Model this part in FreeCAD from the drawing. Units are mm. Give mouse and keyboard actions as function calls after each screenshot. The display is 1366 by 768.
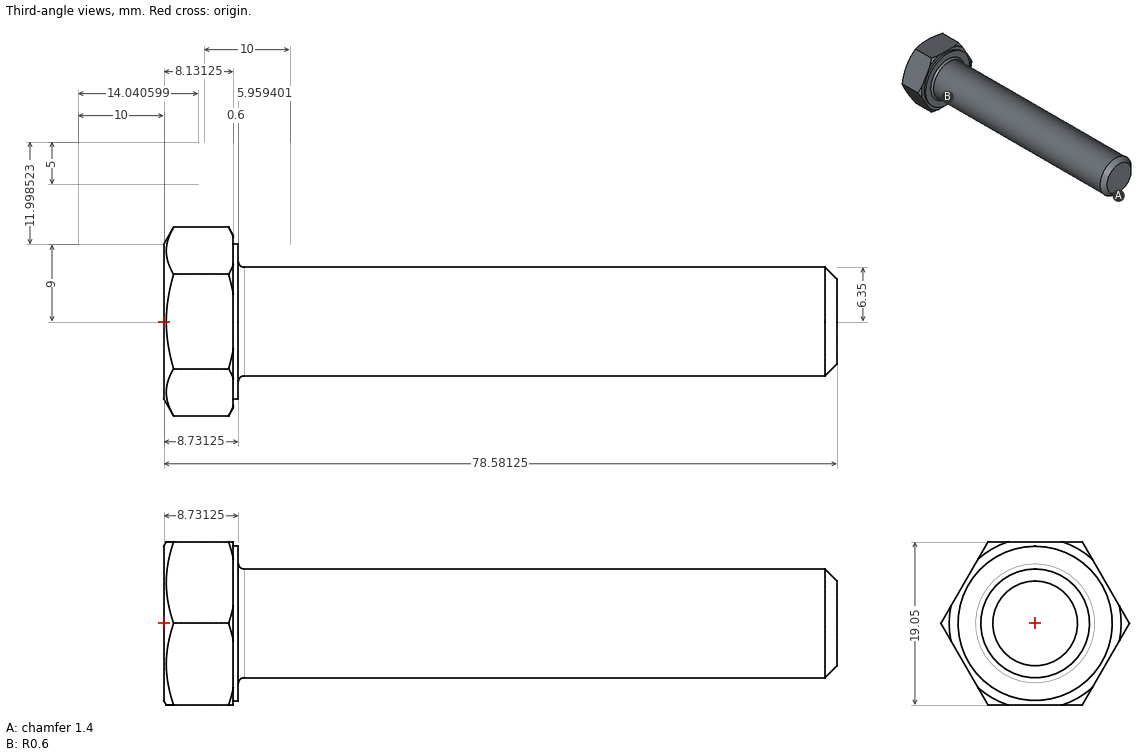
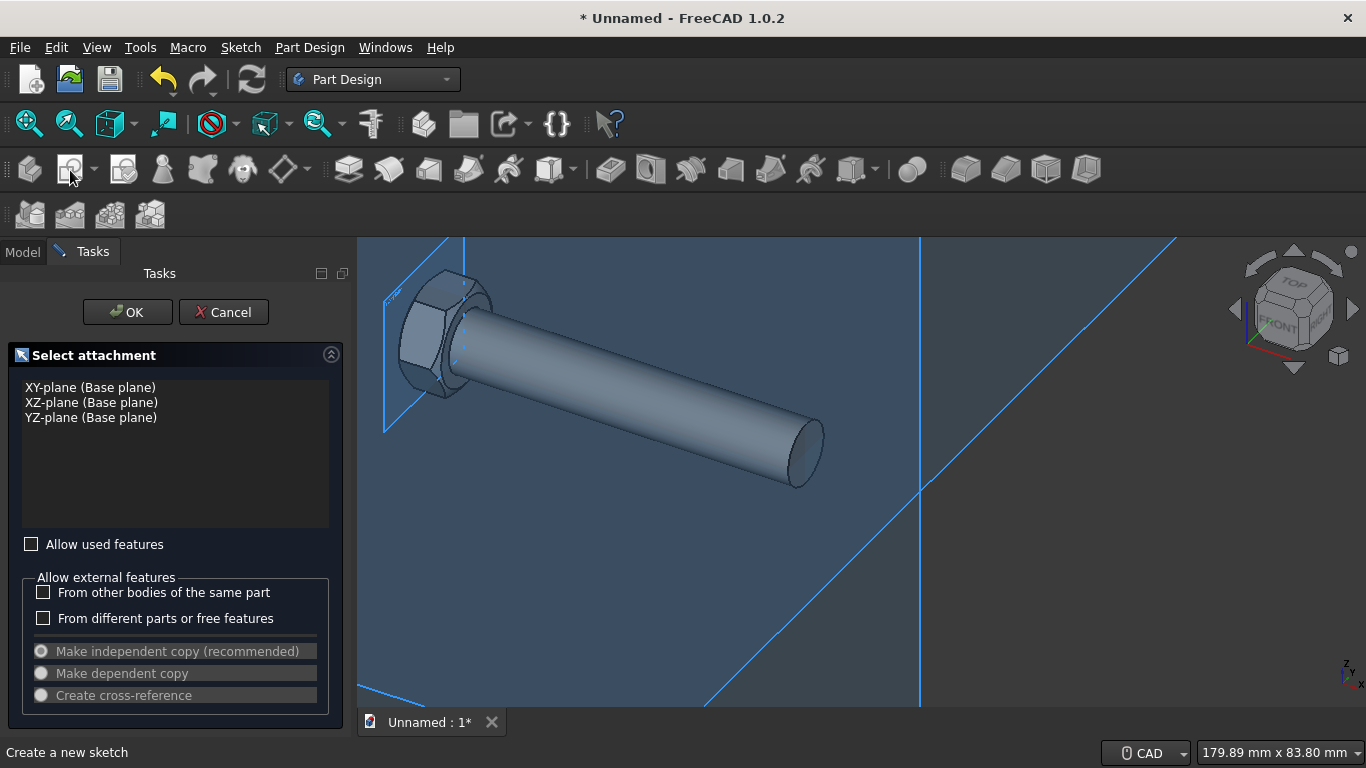
click(82, 388)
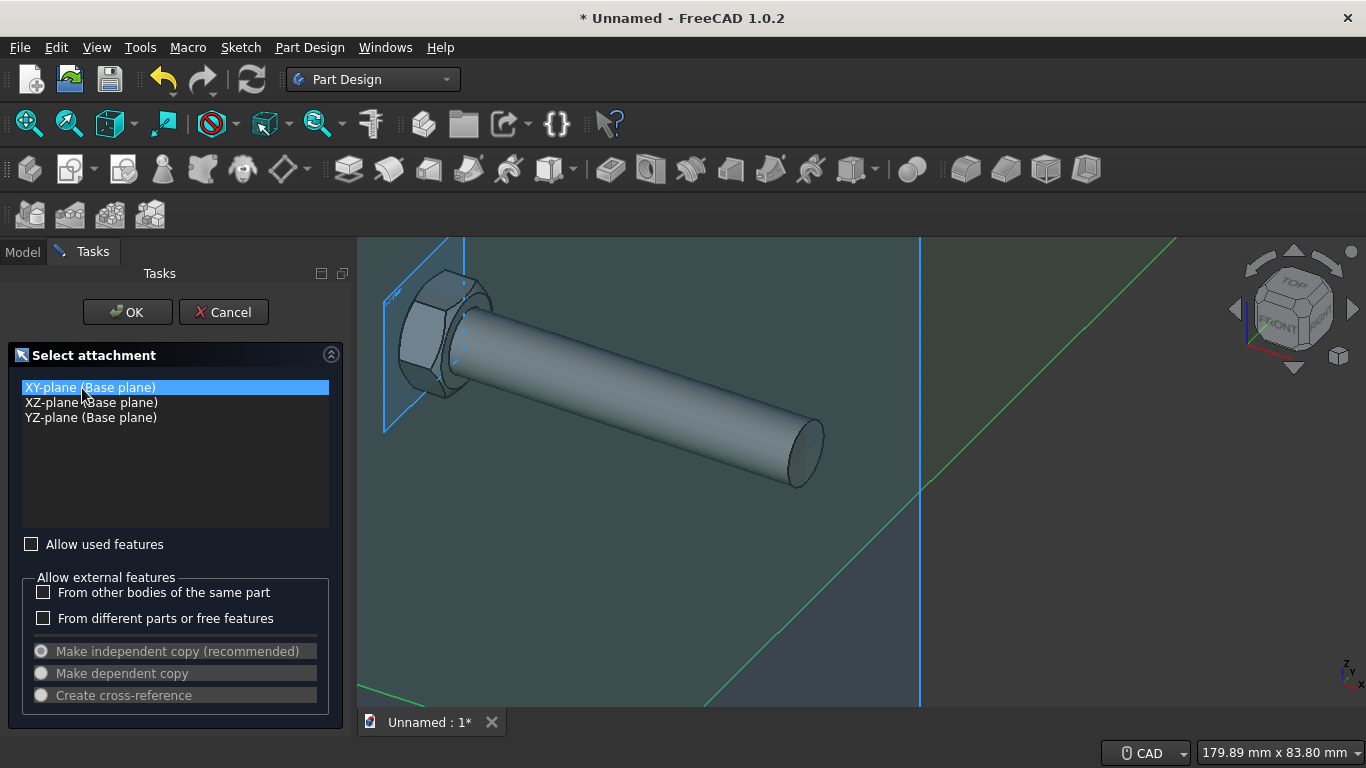
click(128, 312)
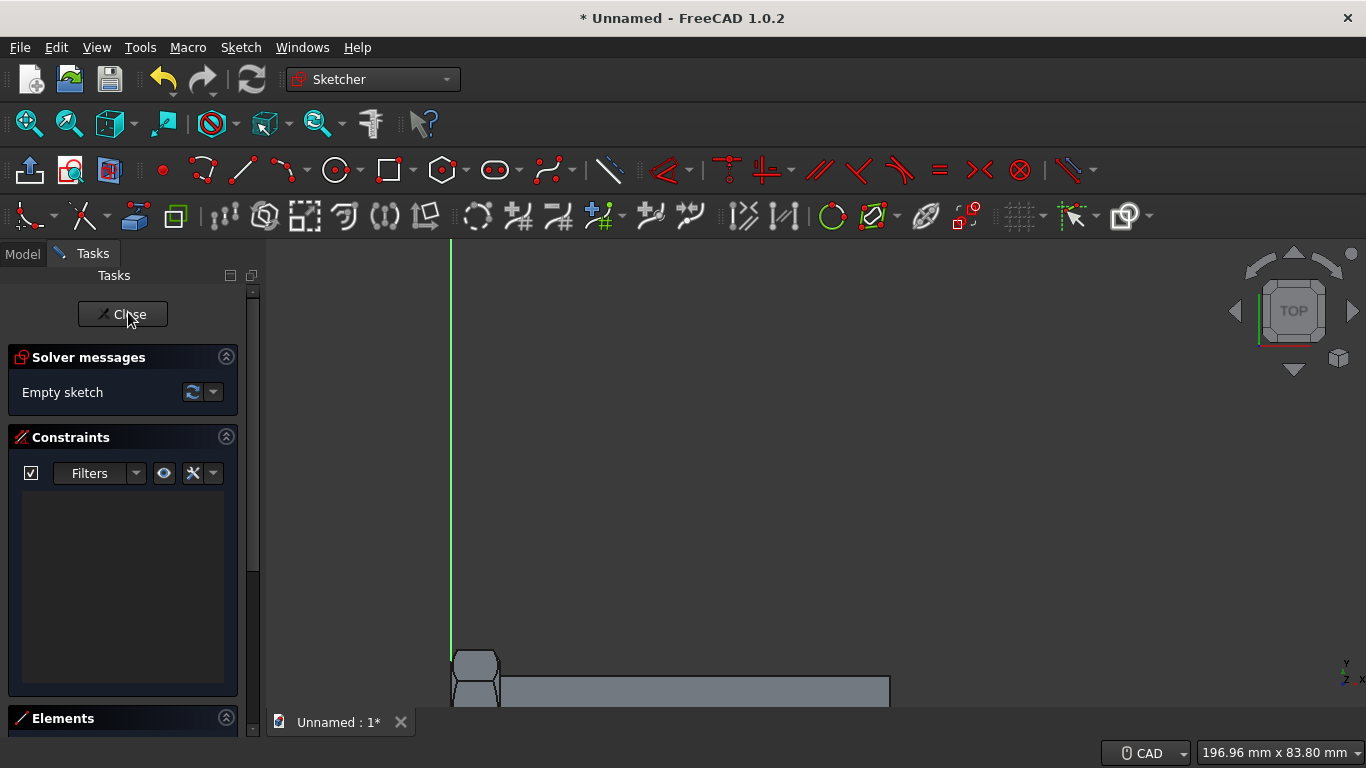
click(110, 170)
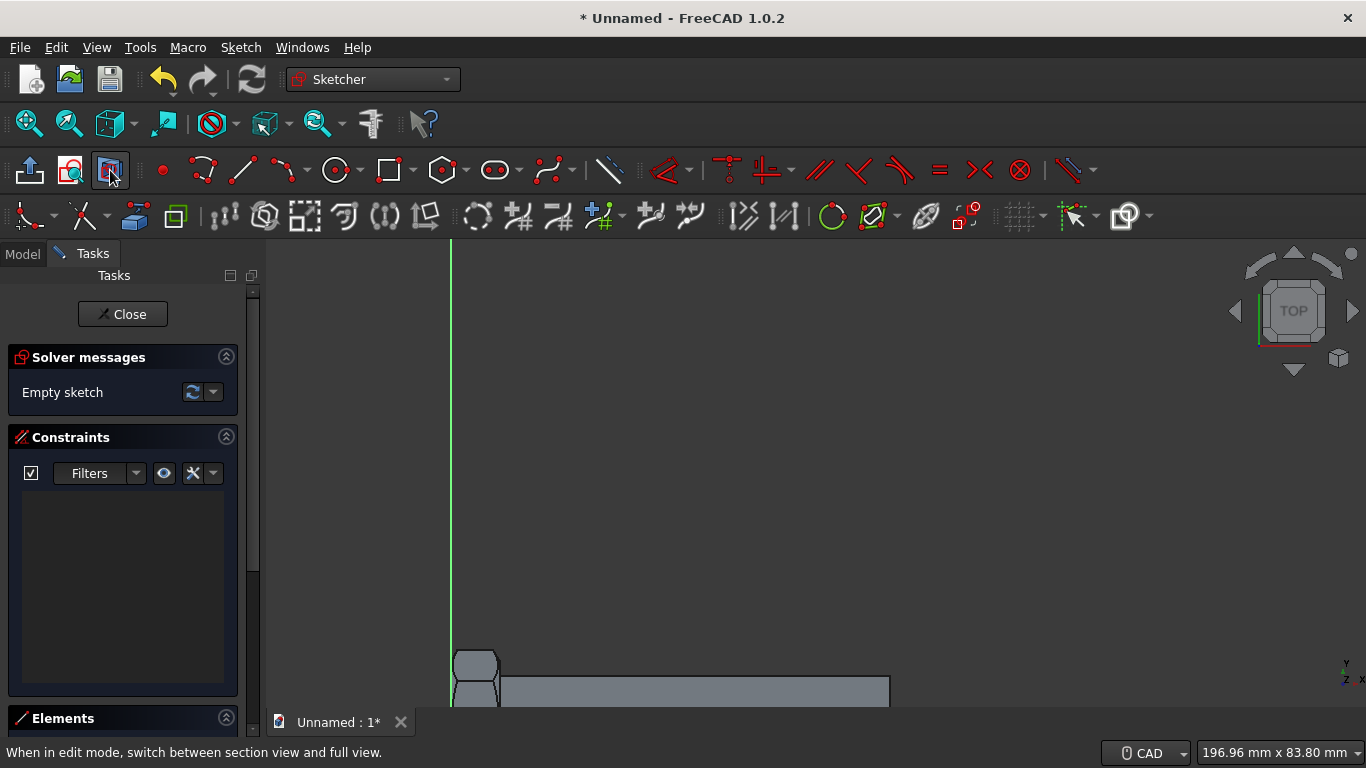
scroll(748, 473, down, 5)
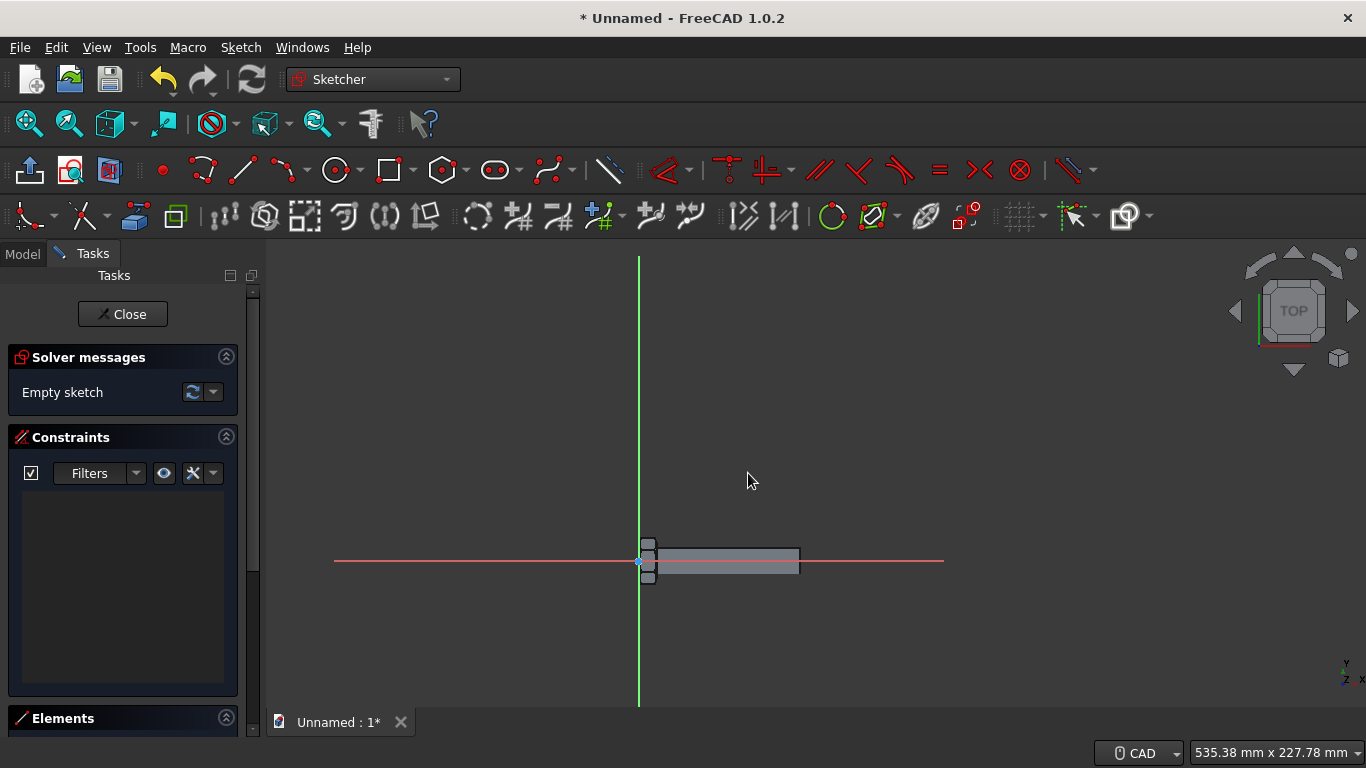
scroll(632, 550, up, 10)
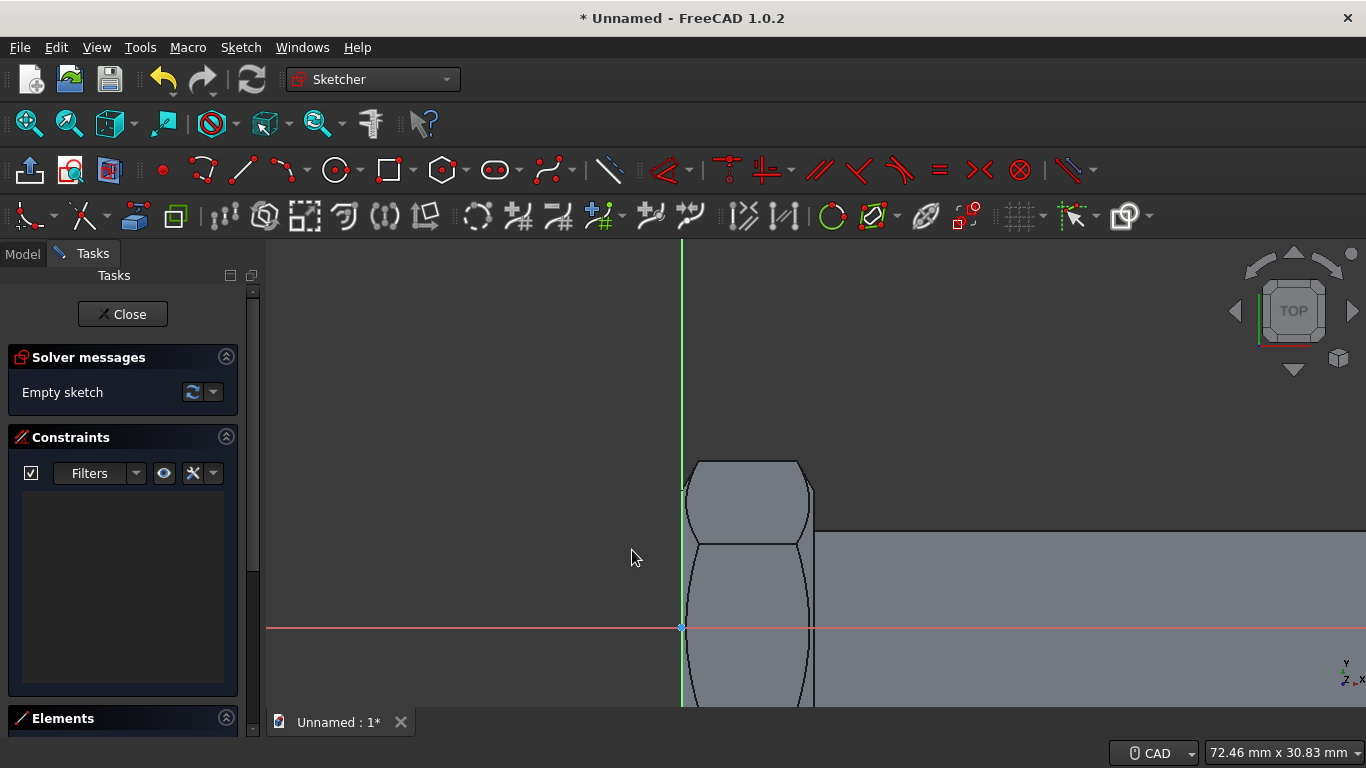
click(390, 170)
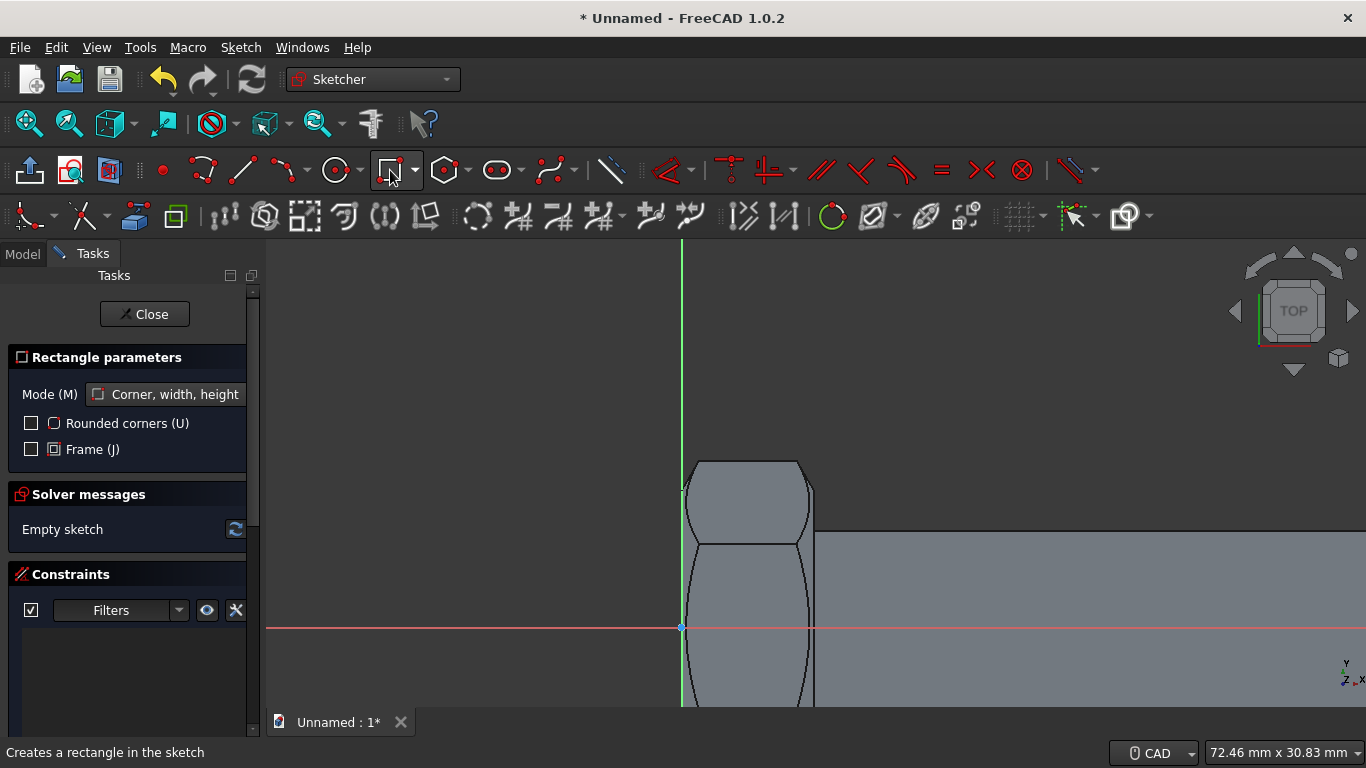
scroll(805, 309, up, 3)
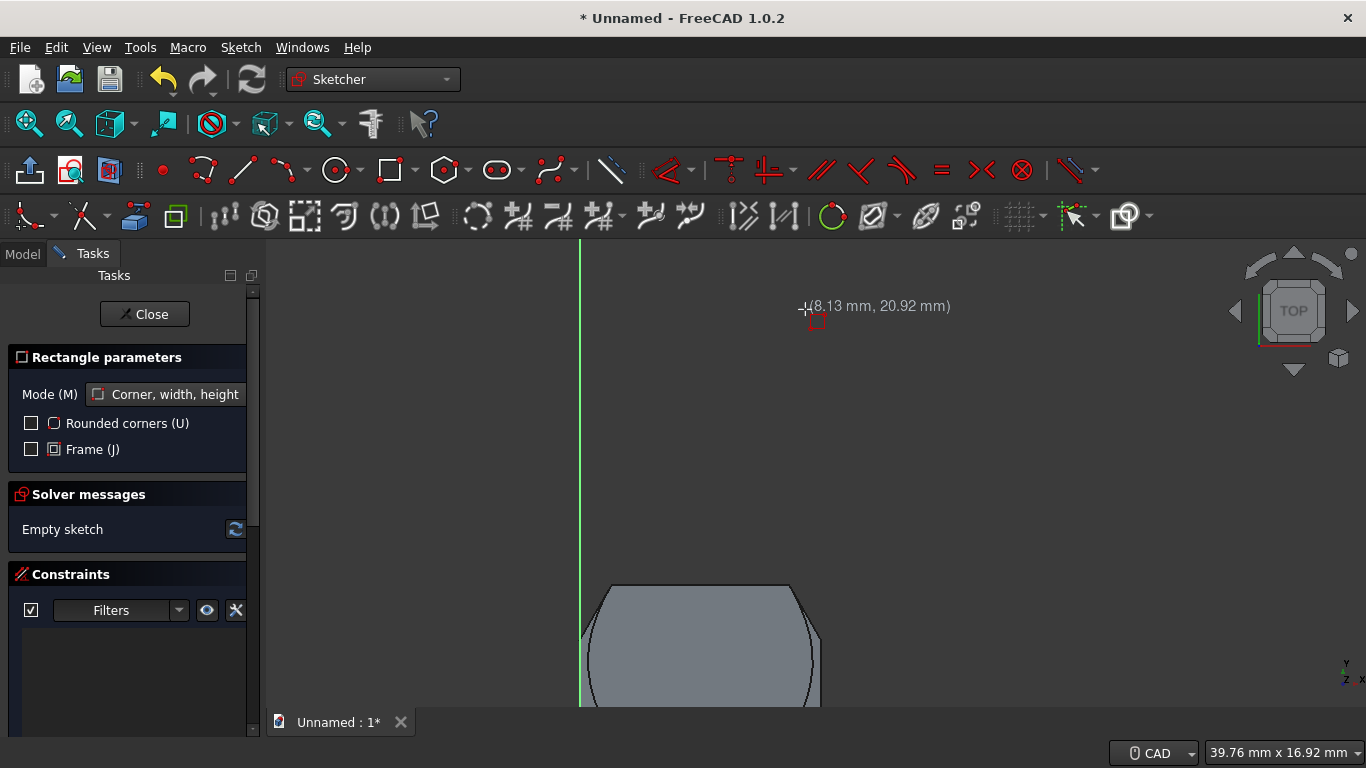
click(805, 308)
move(821, 640)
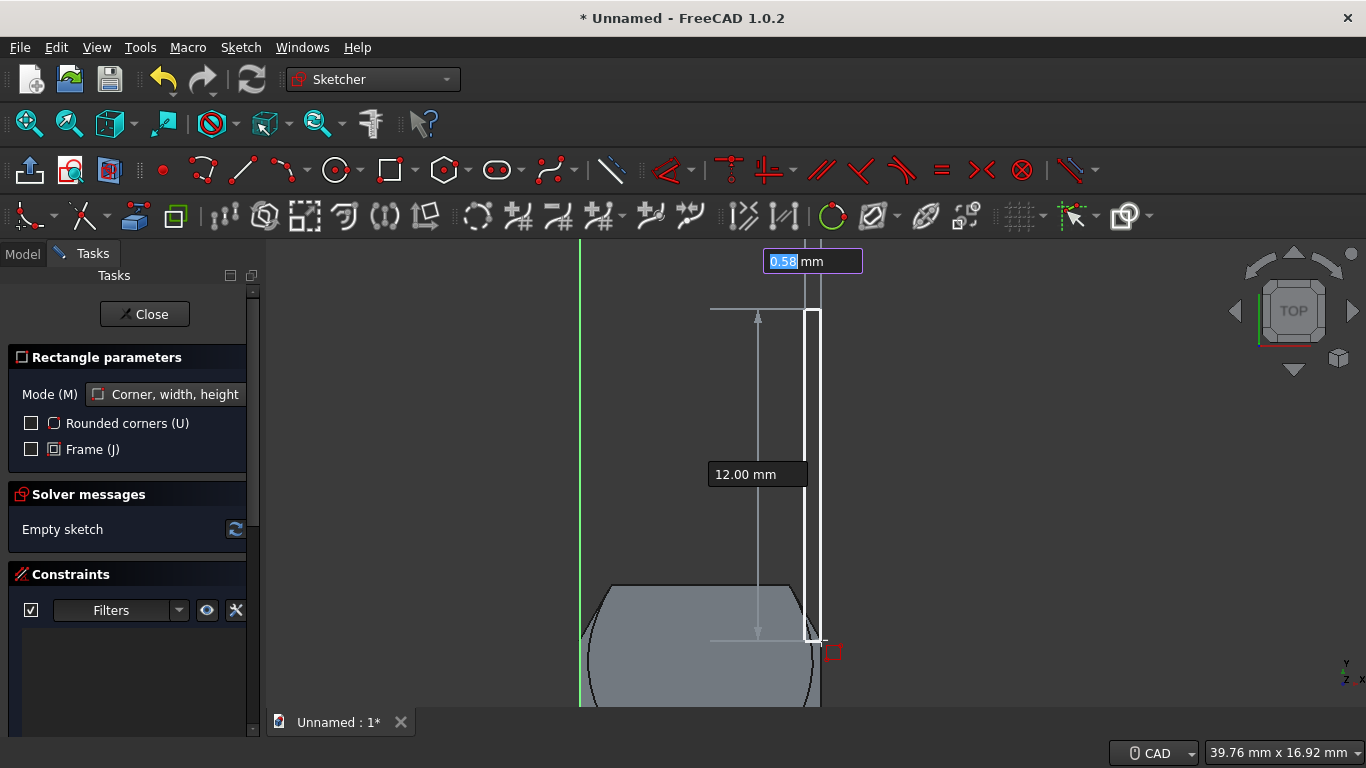
text(0.6)
key(Tab)
text(11.998523)
key(Return)
key(Escape)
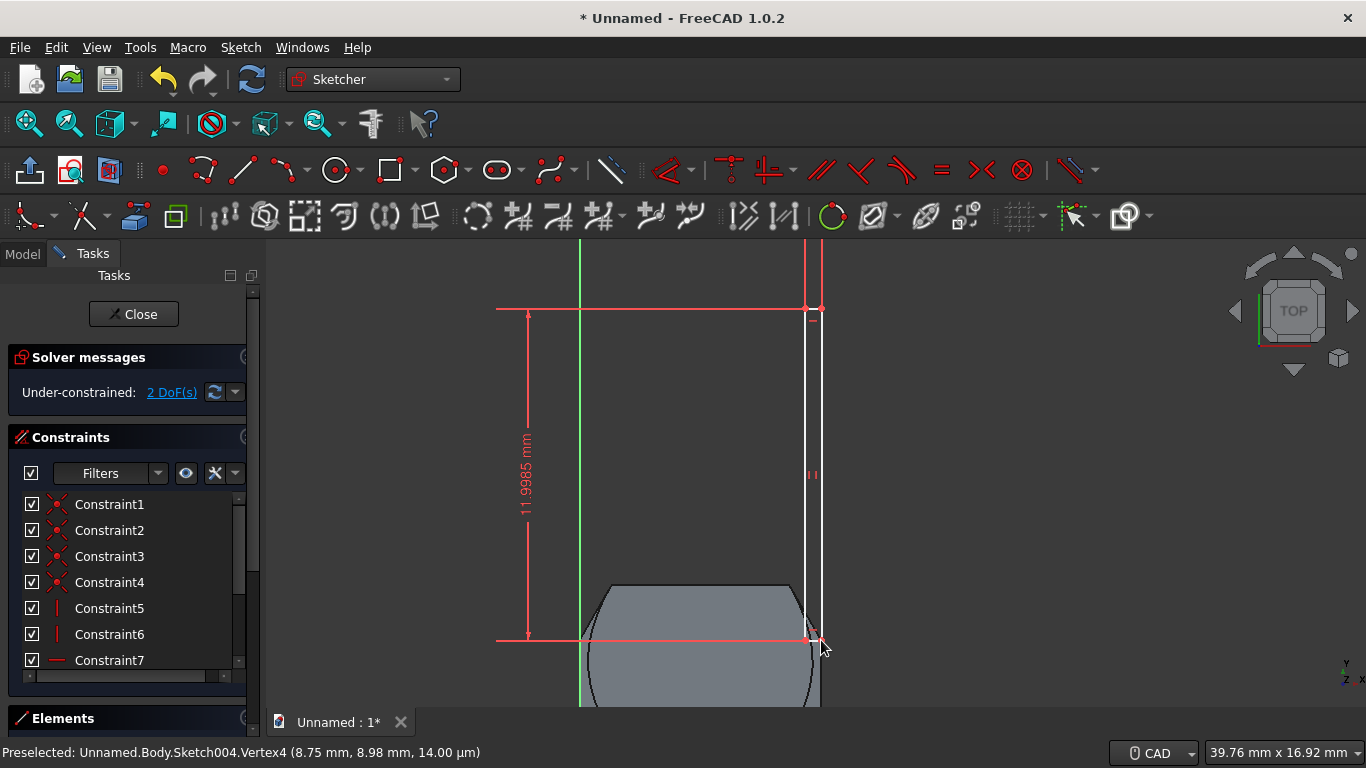
click(666, 170)